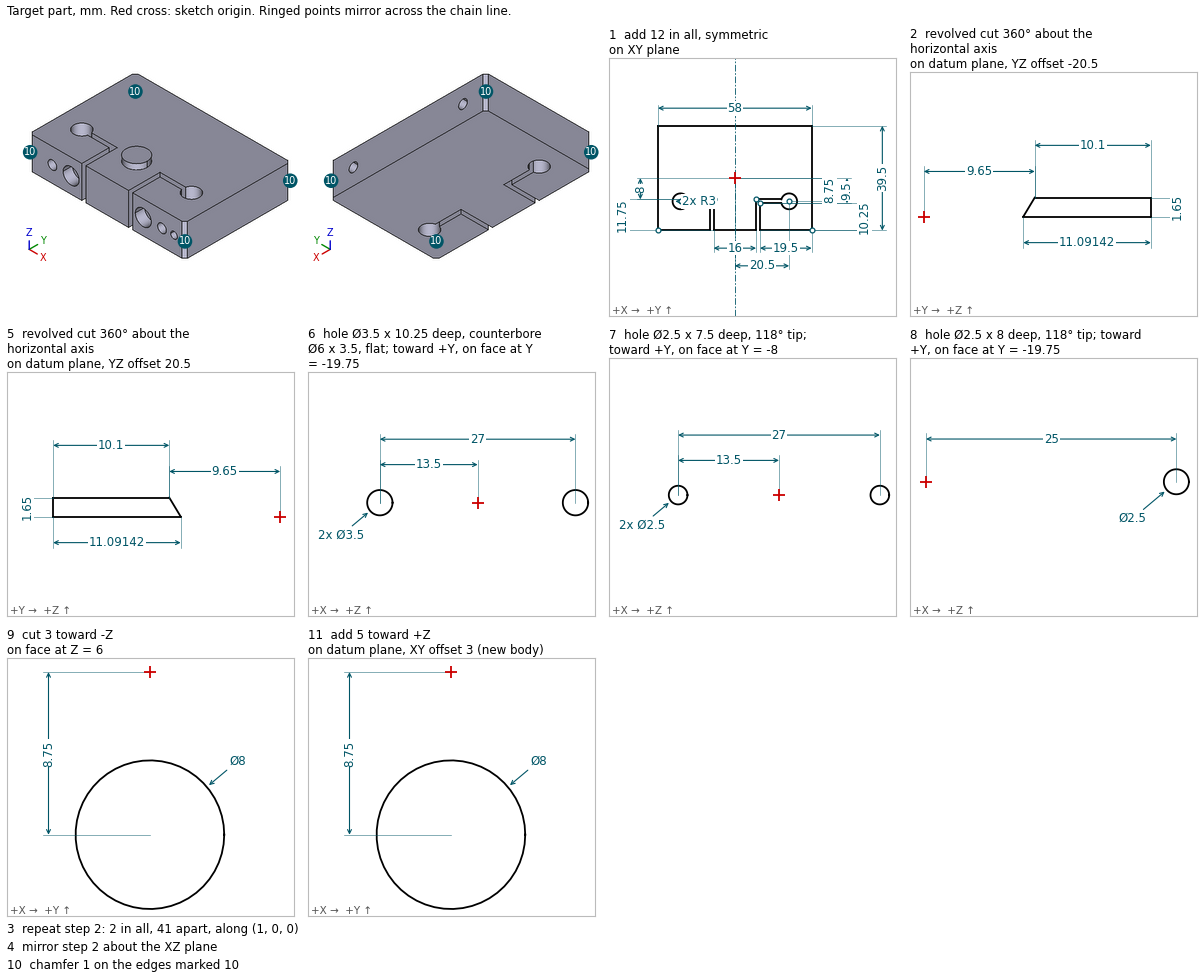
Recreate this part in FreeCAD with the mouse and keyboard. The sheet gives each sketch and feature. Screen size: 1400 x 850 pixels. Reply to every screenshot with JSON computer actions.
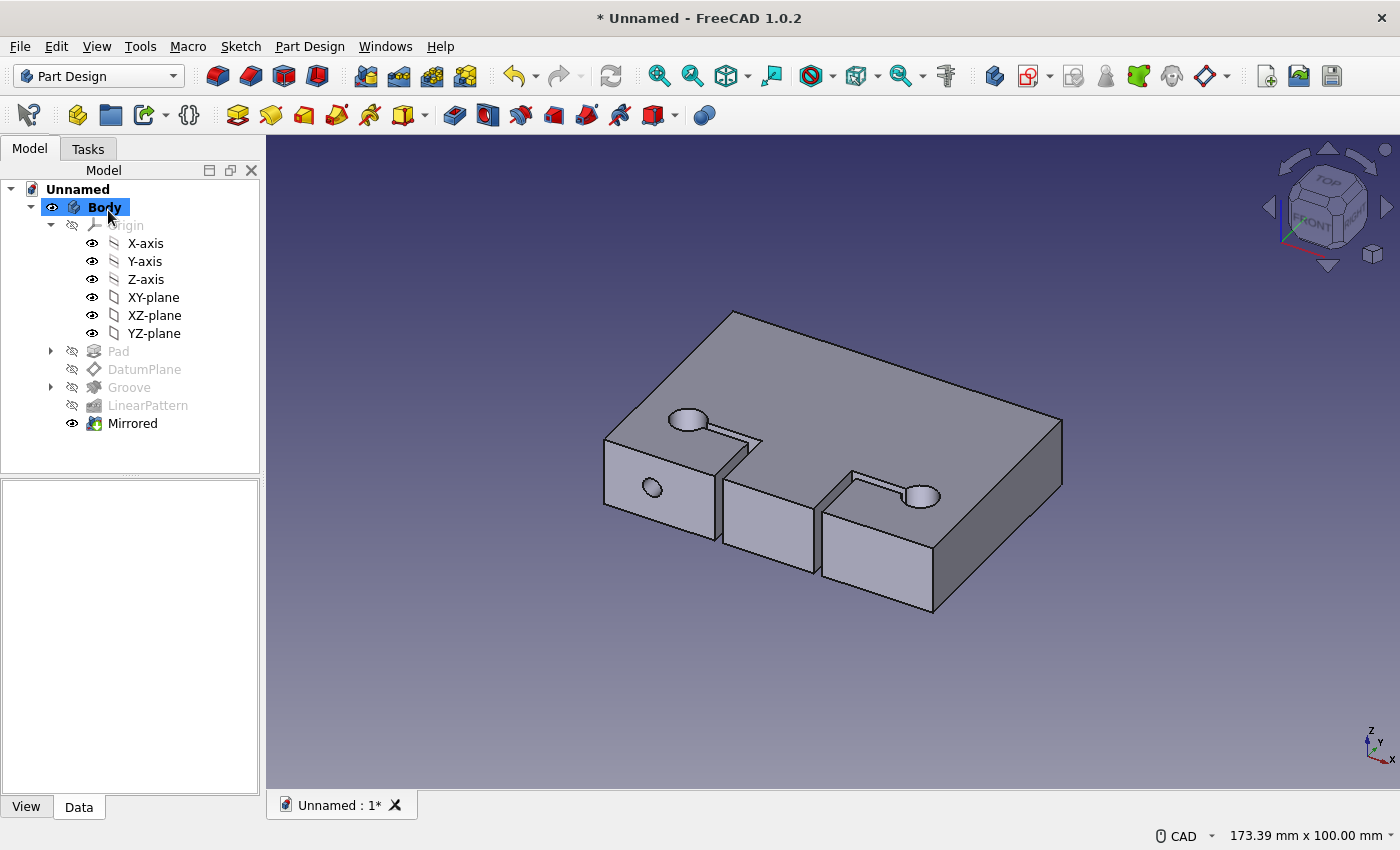
{"action": "left_click", "coordinate": [137, 333]}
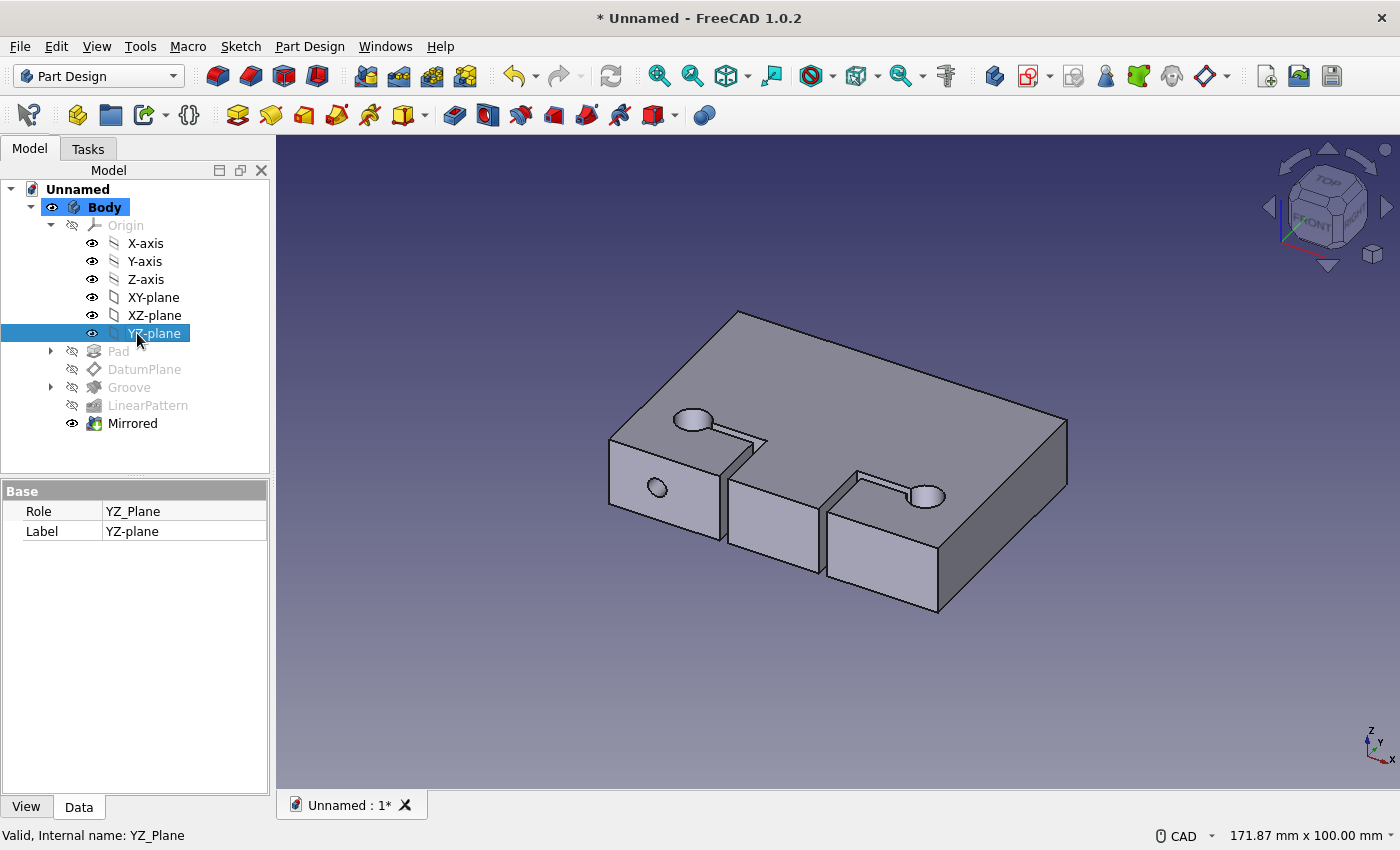
{"action": "left_click", "coordinate": [1204, 76]}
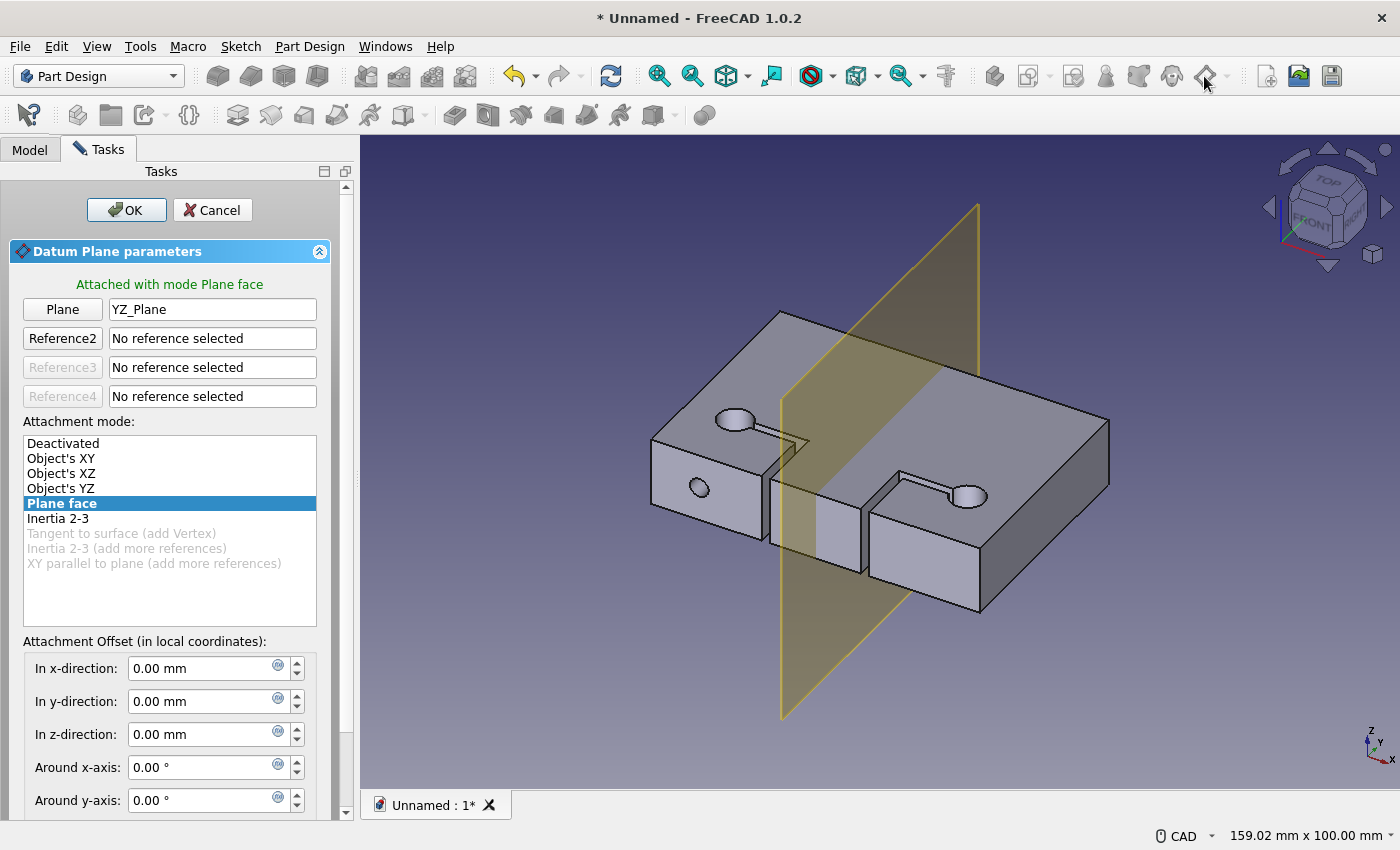
{"action": "triple_click", "coordinate": [210, 734]}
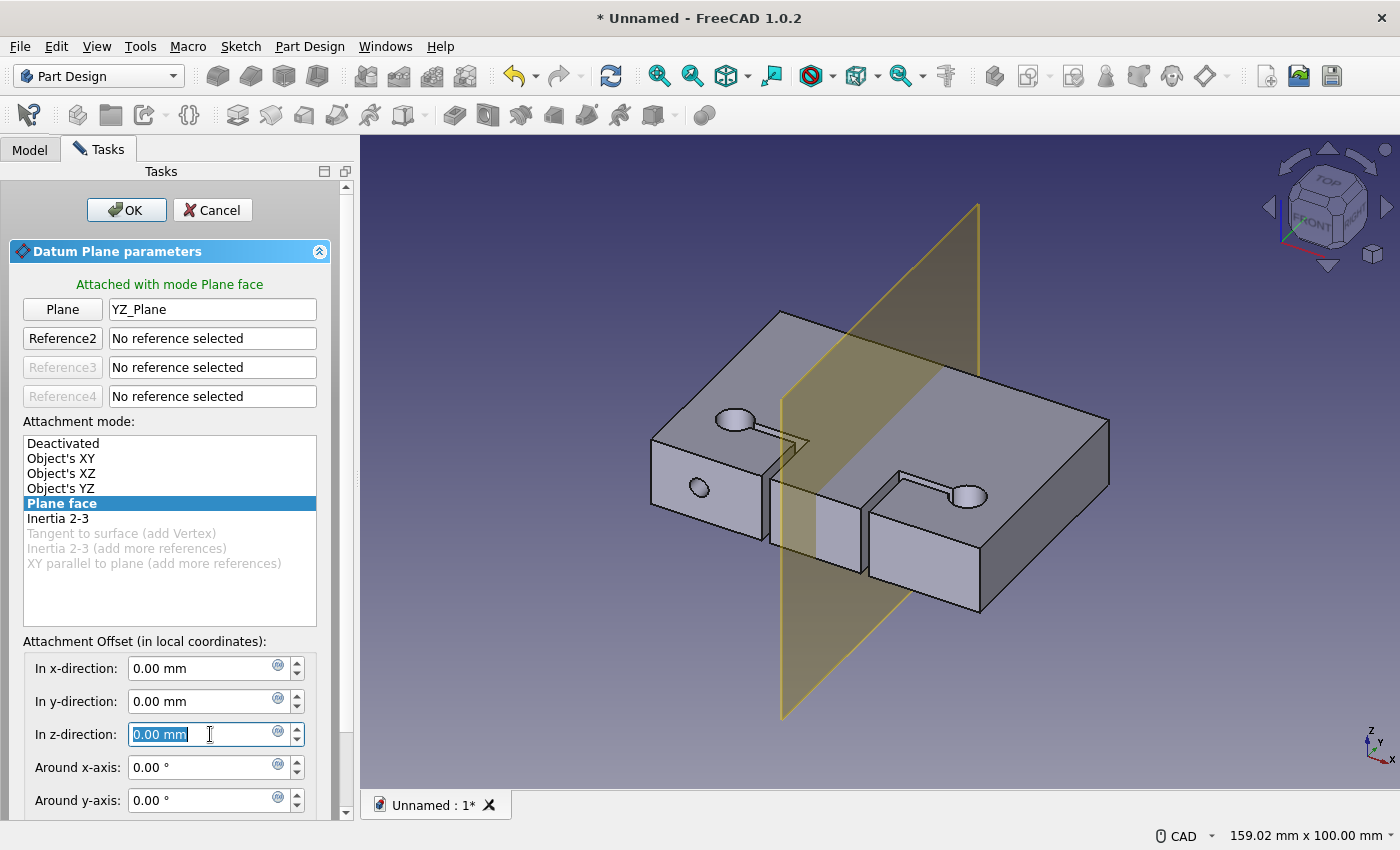
{"action": "type", "text": "20.5"}
{"action": "key", "text": "Tab"}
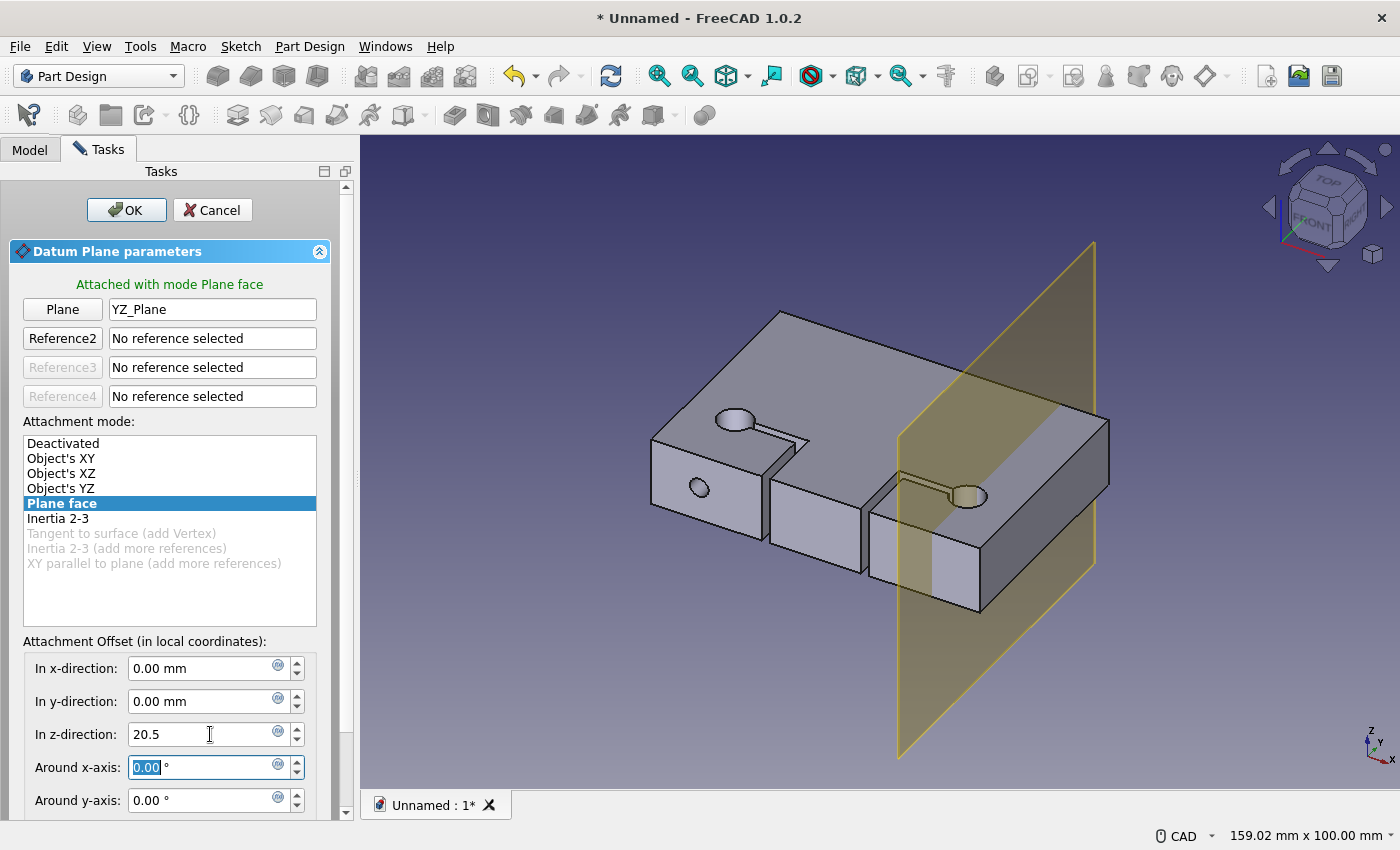
{"action": "left_click", "coordinate": [127, 210]}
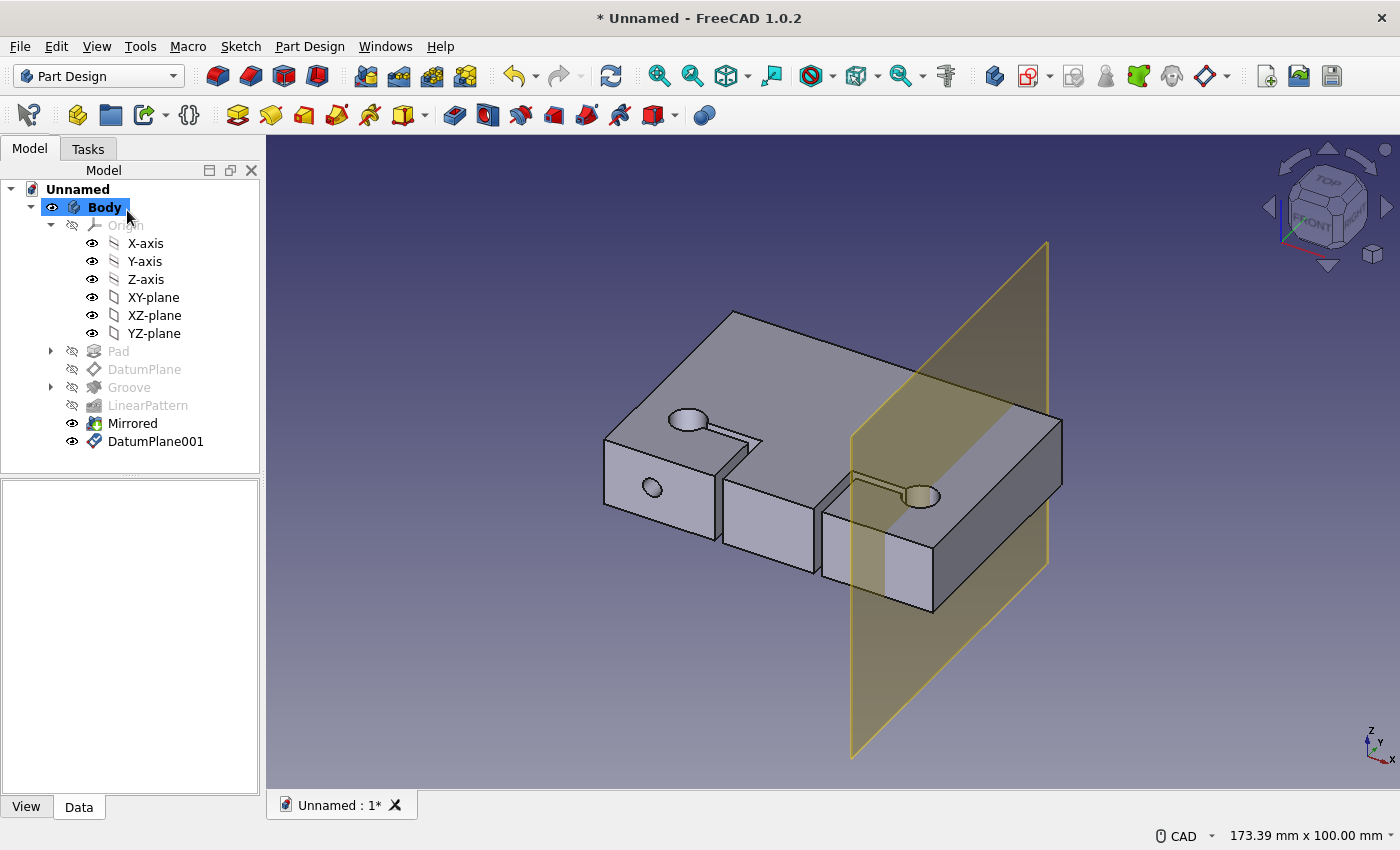
{"action": "left_click", "coordinate": [117, 441]}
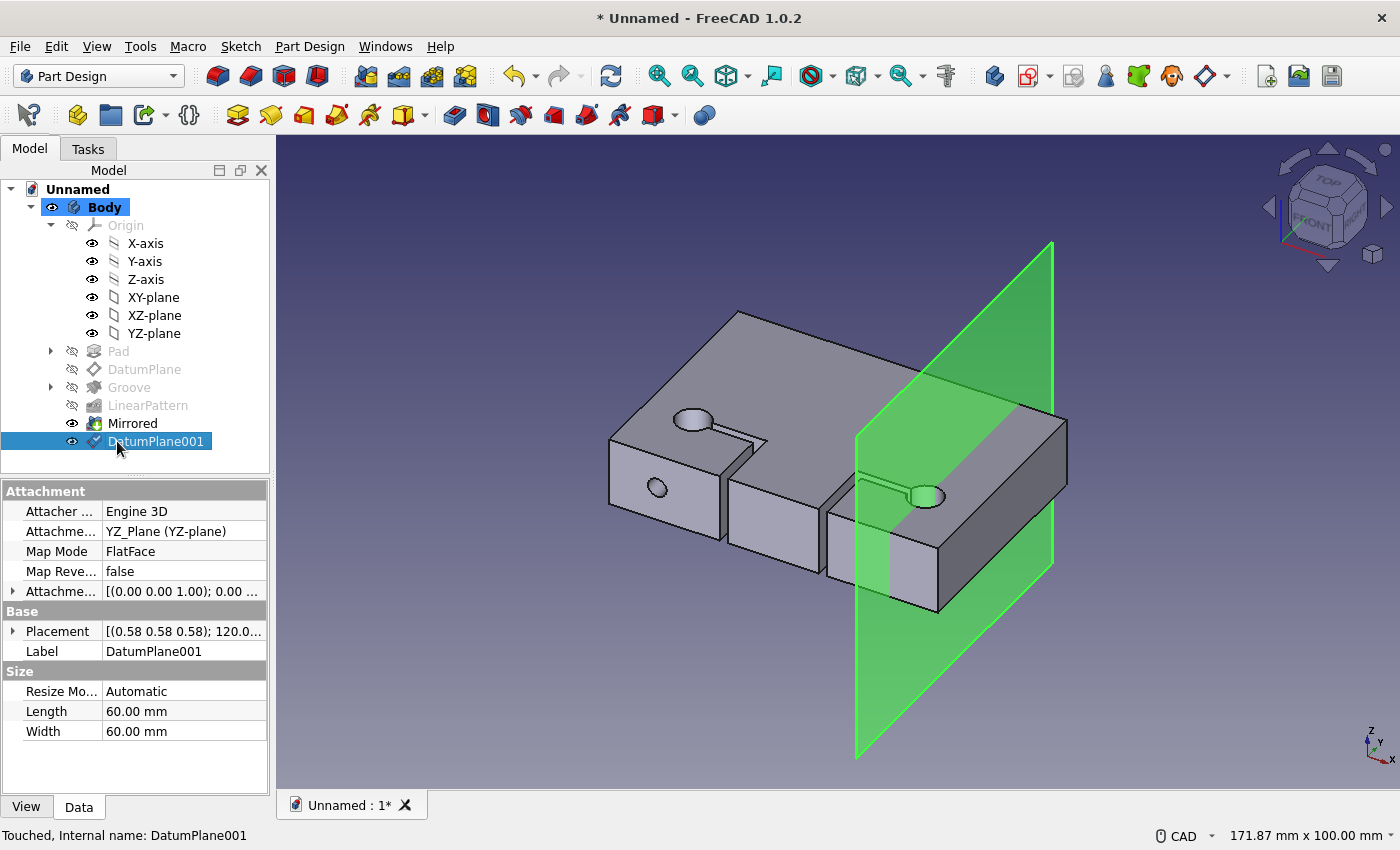
{"action": "left_click", "coordinate": [1028, 76]}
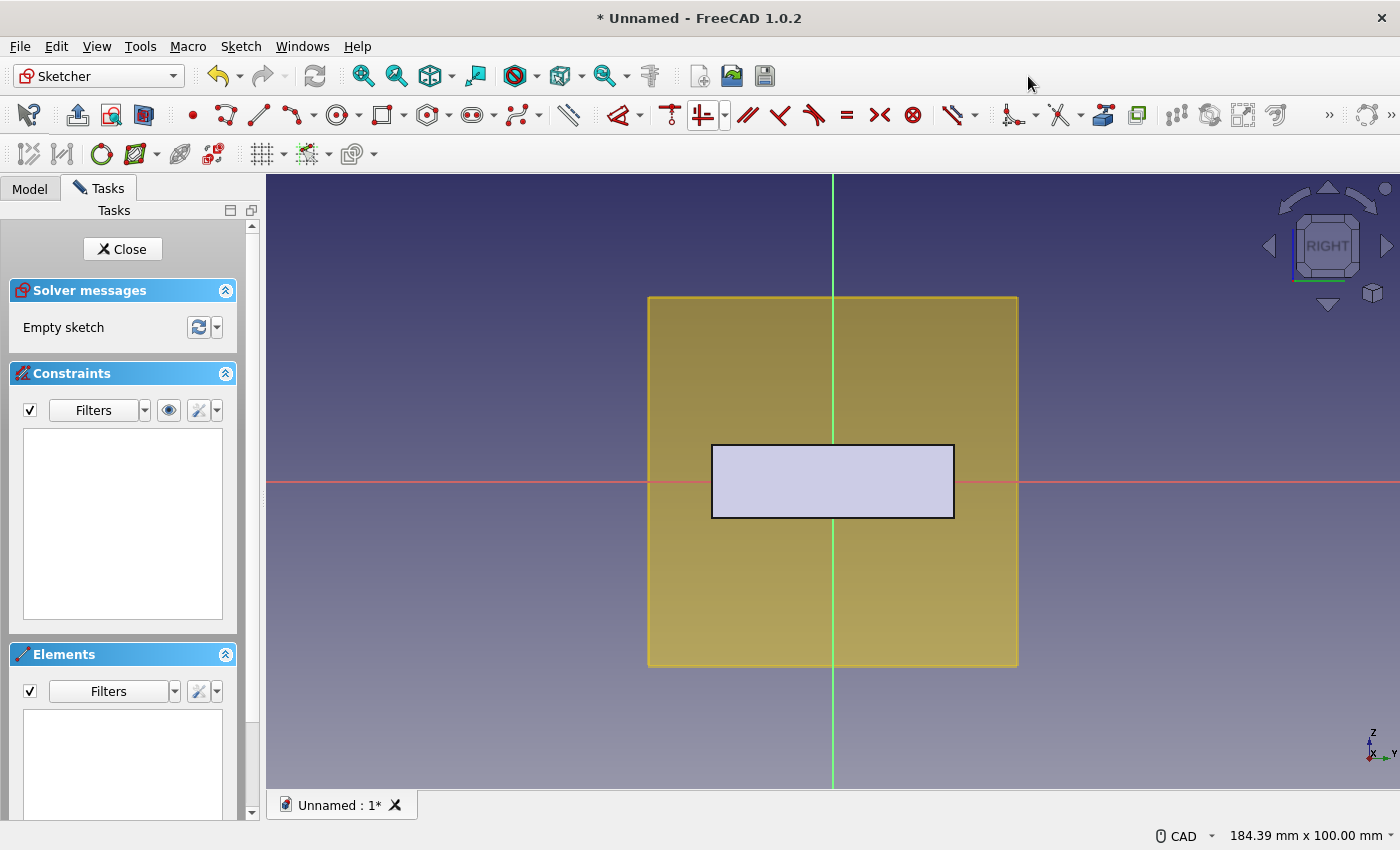
{"action": "left_click", "coordinate": [144, 116]}